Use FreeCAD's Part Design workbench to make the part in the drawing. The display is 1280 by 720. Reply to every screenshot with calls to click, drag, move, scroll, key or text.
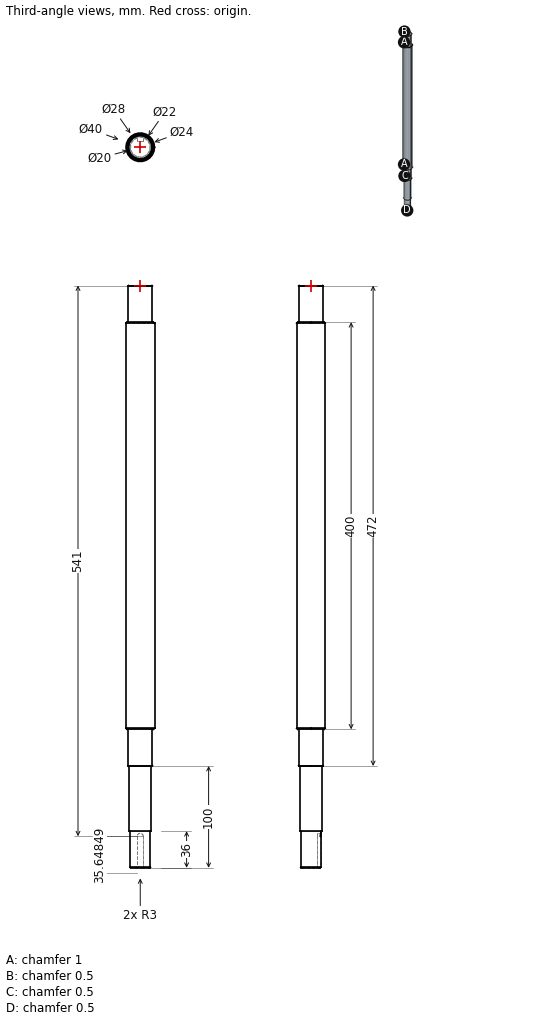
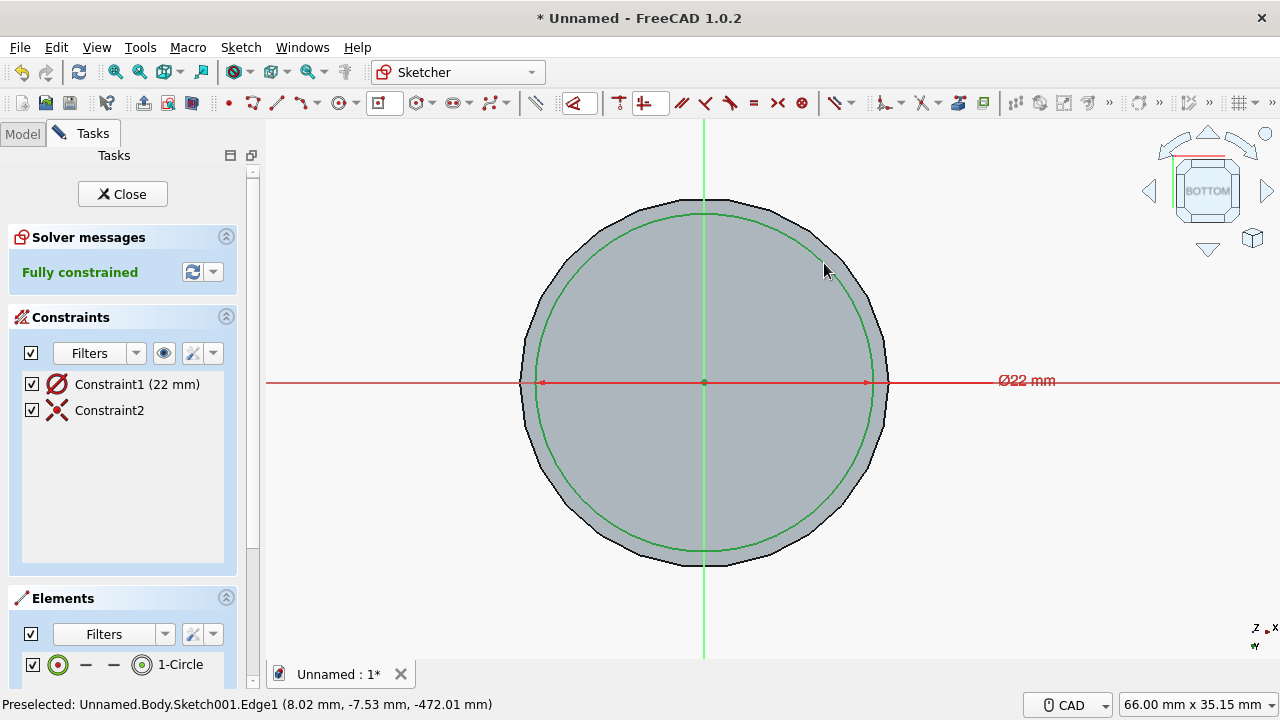
click(123, 194)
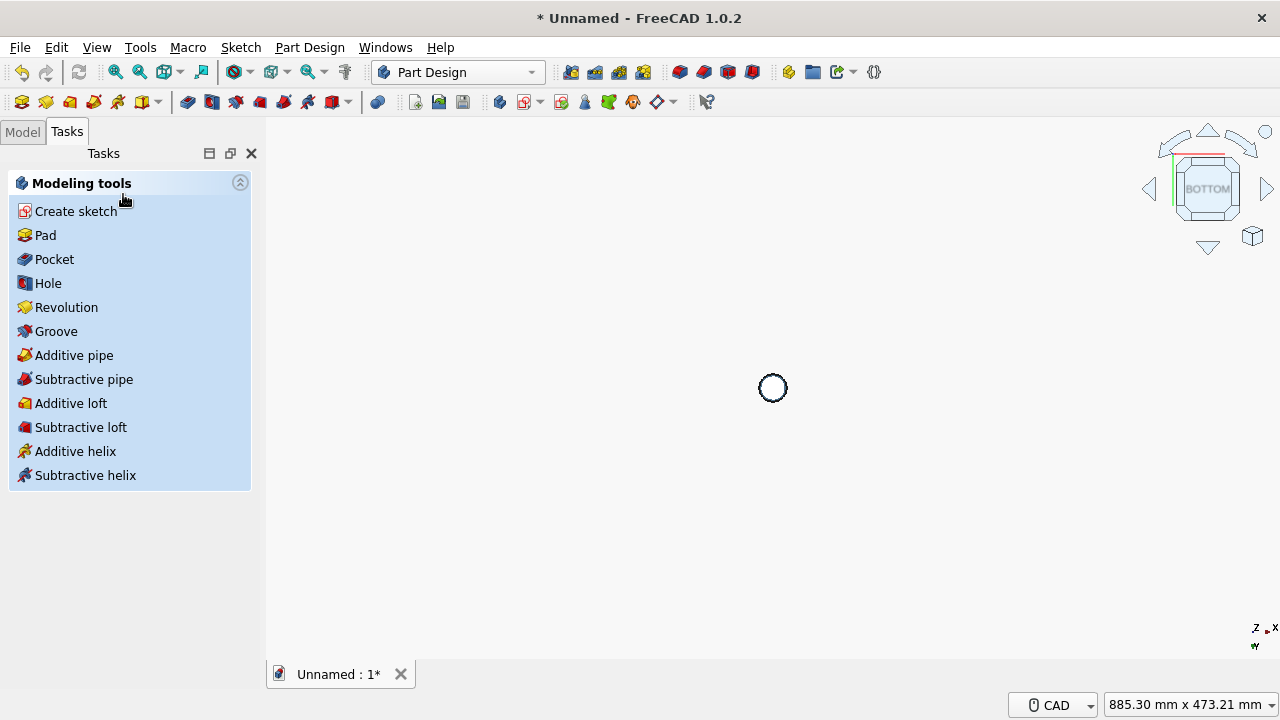
click(22, 102)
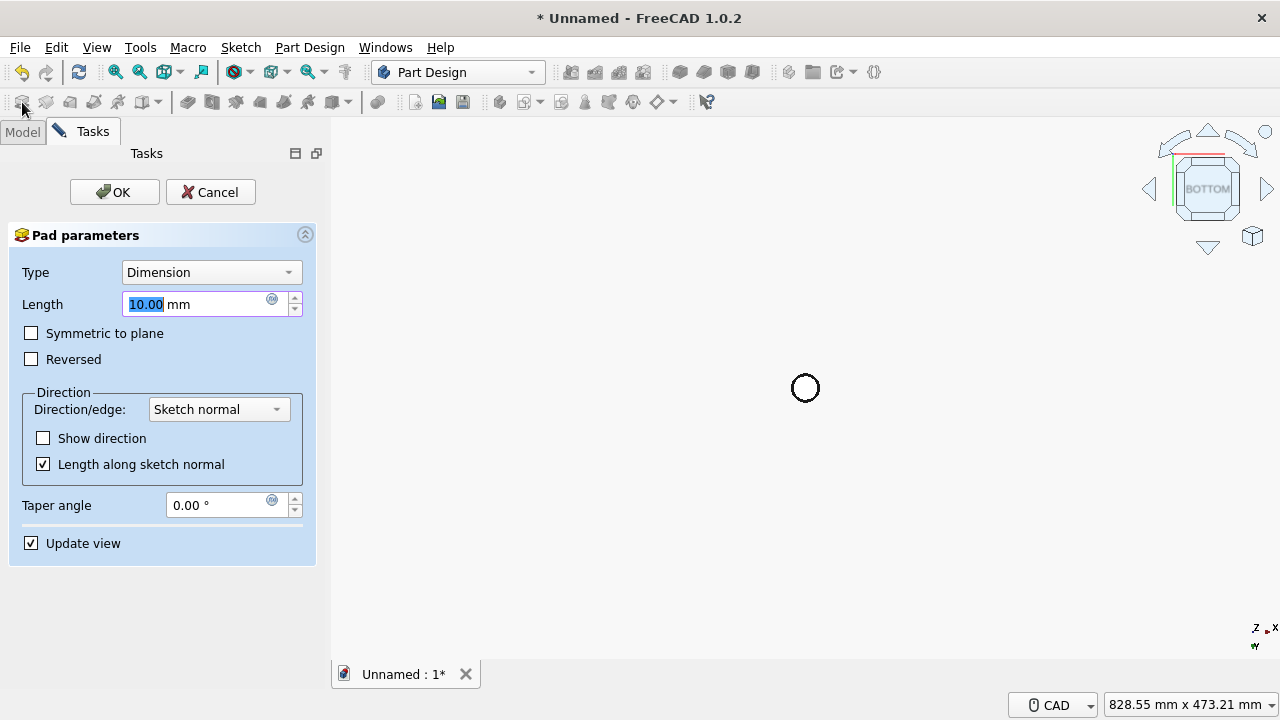
text(100)
key(Tab)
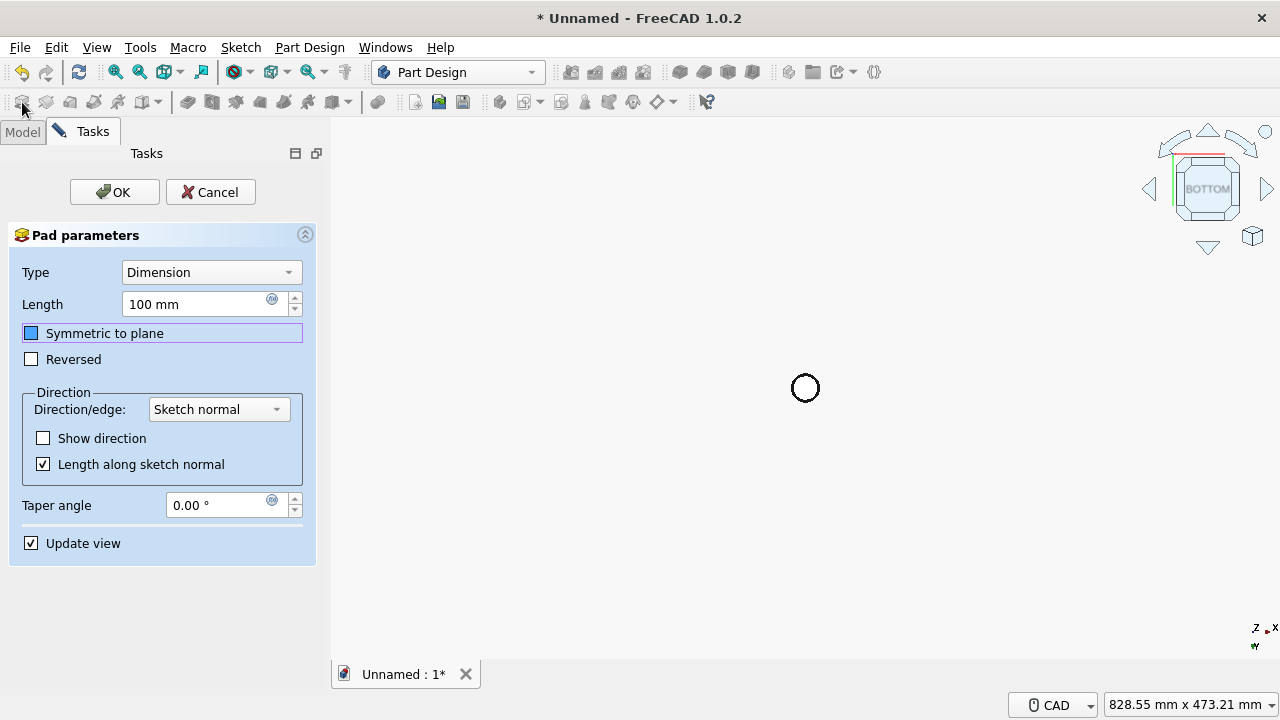
click(115, 192)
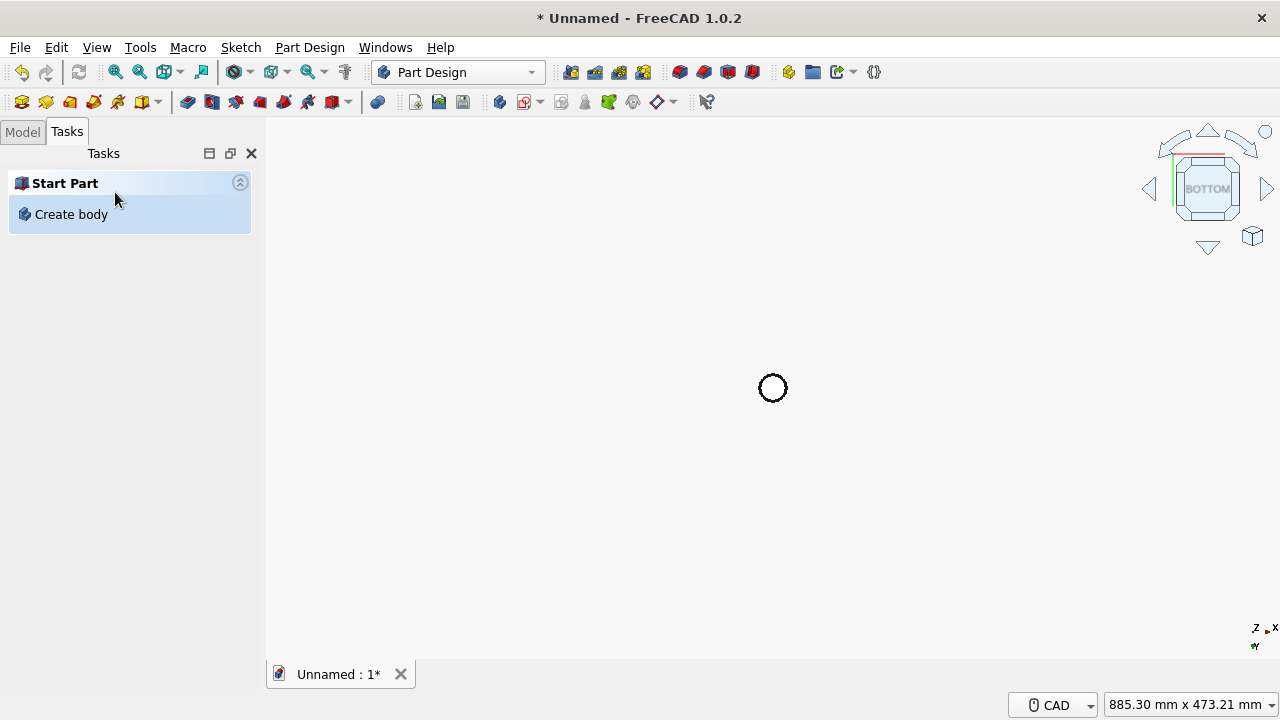
click(116, 72)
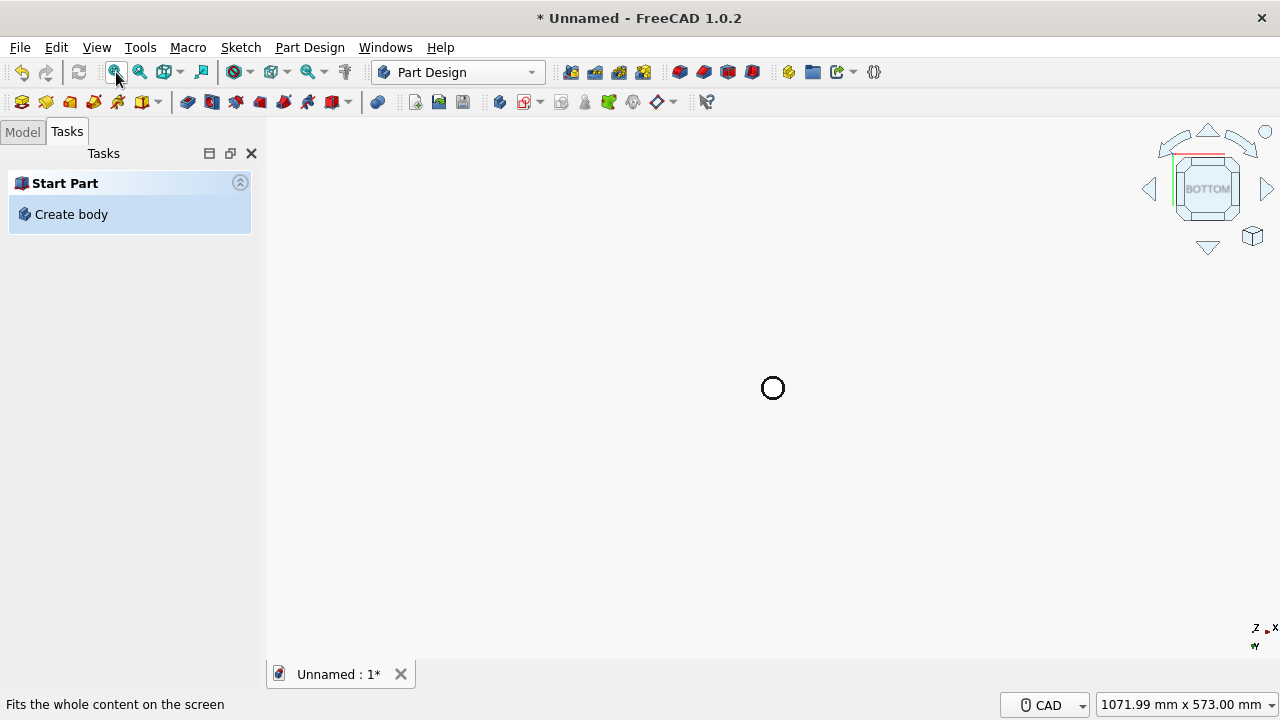
click(23, 131)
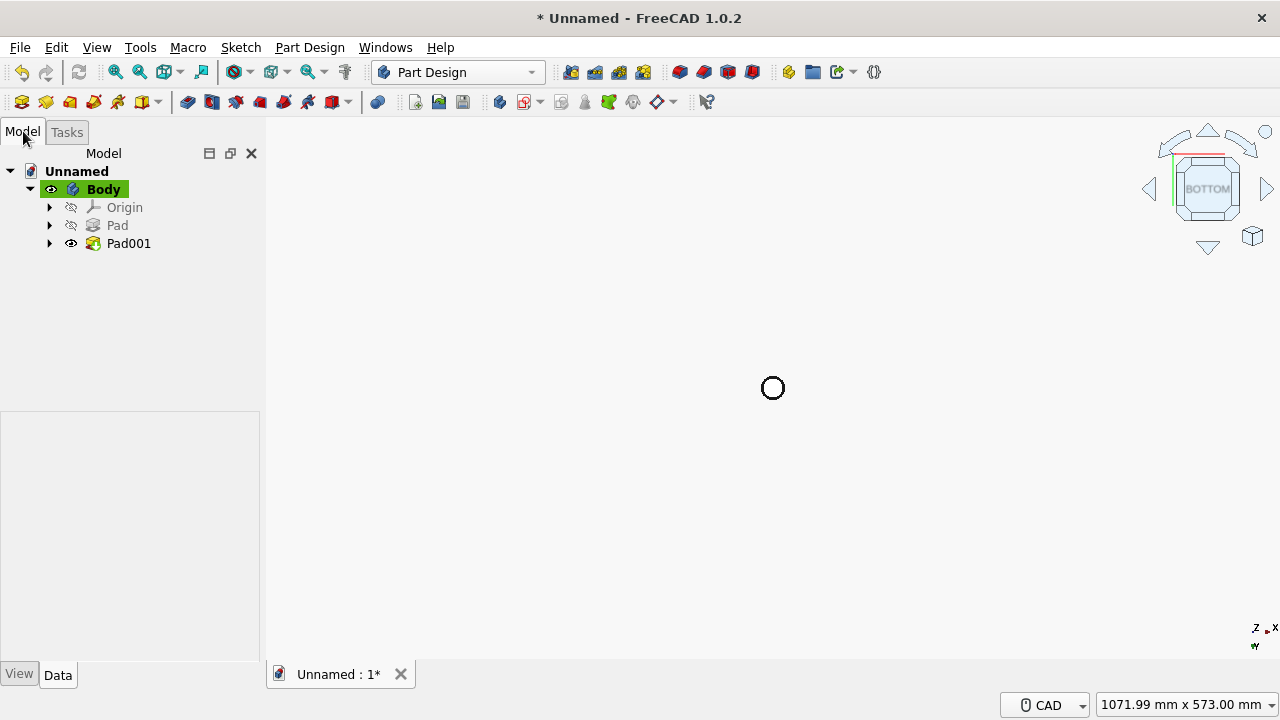
click(50, 207)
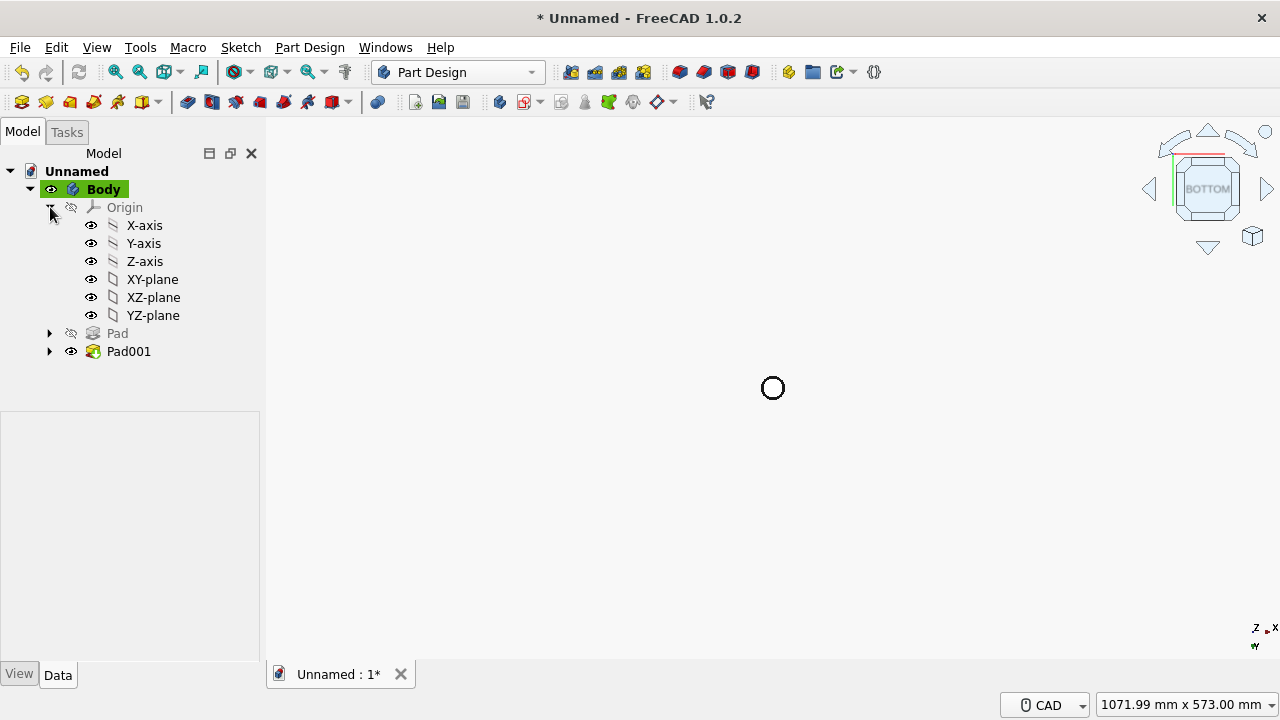
click(136, 279)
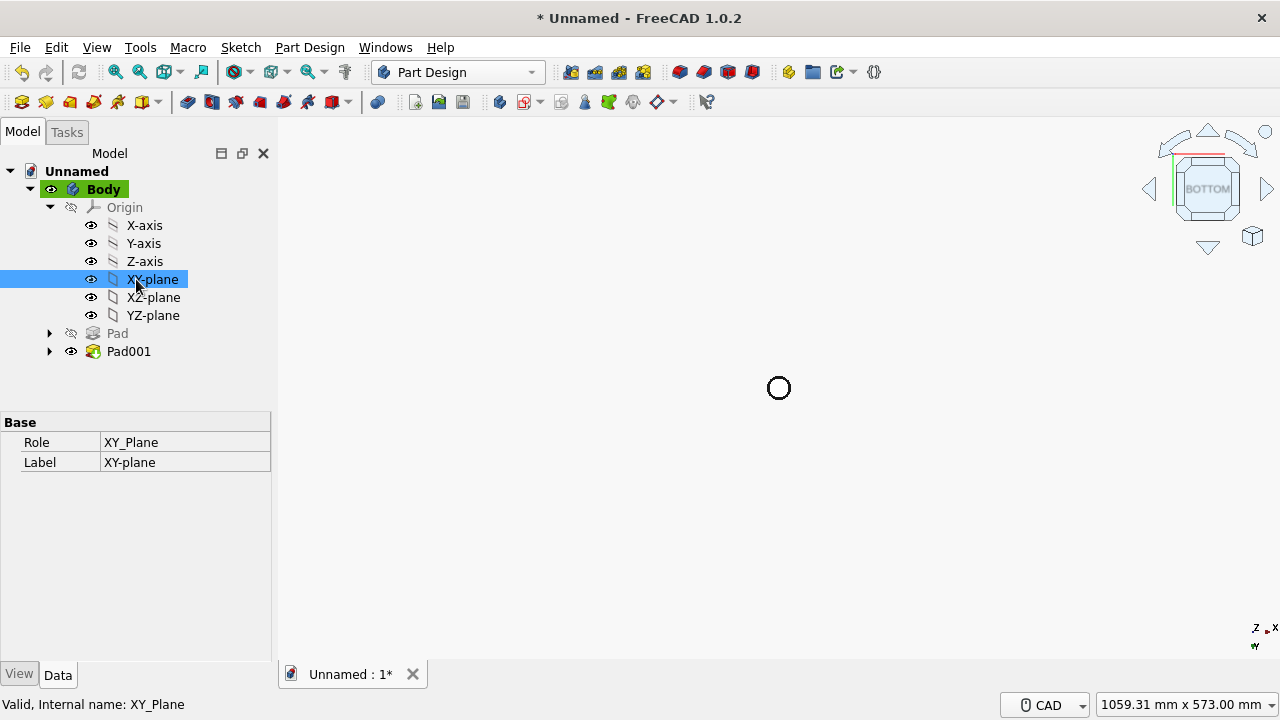
click(658, 102)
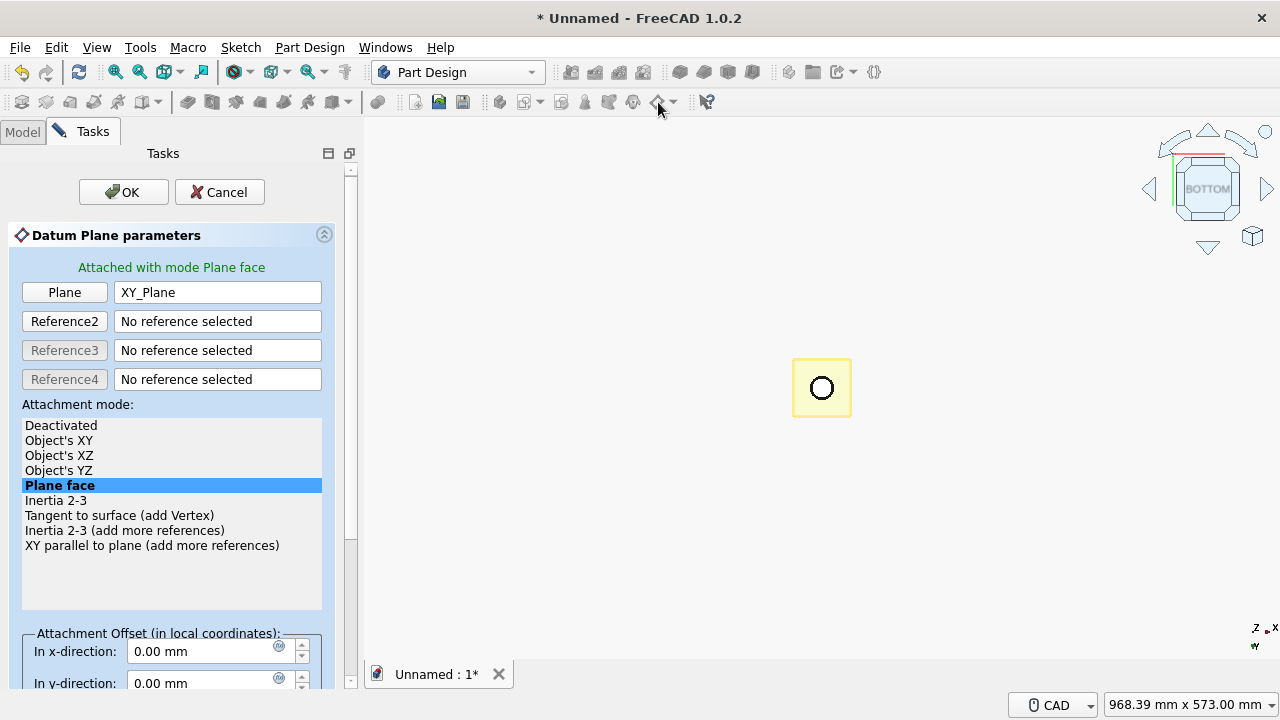
scroll(351, 426, down, 2)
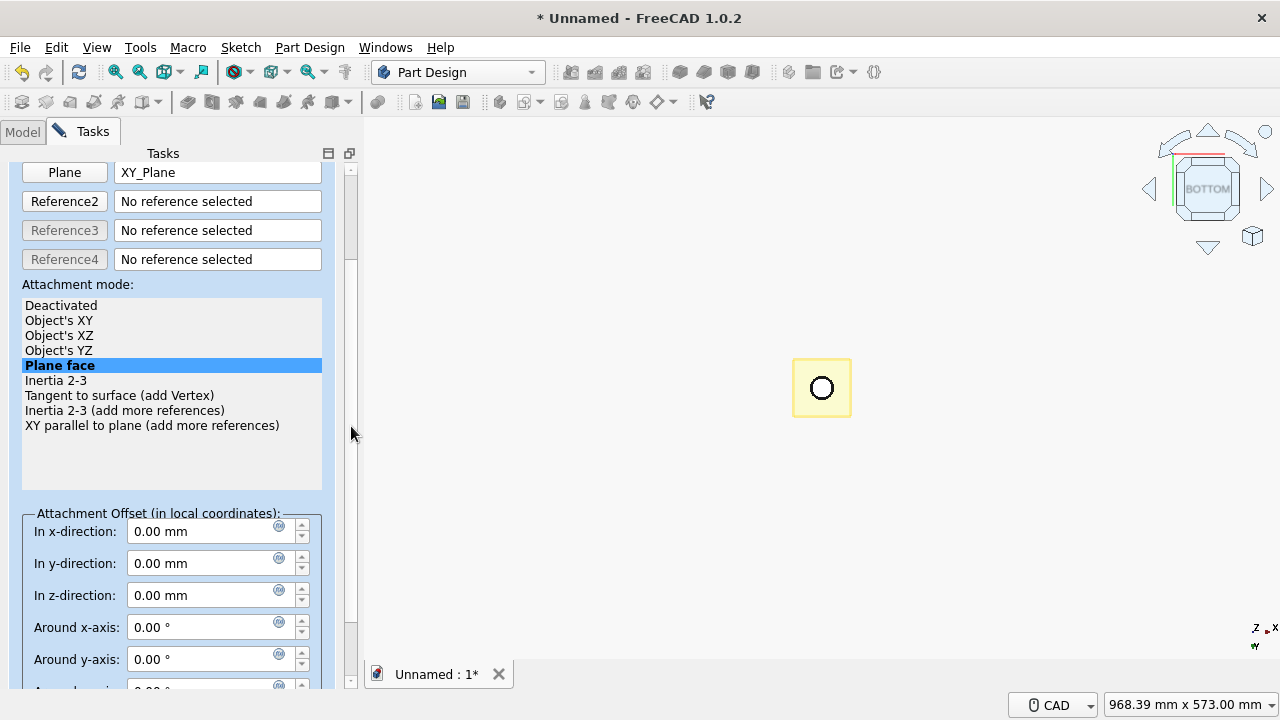
triple_click(210, 595)